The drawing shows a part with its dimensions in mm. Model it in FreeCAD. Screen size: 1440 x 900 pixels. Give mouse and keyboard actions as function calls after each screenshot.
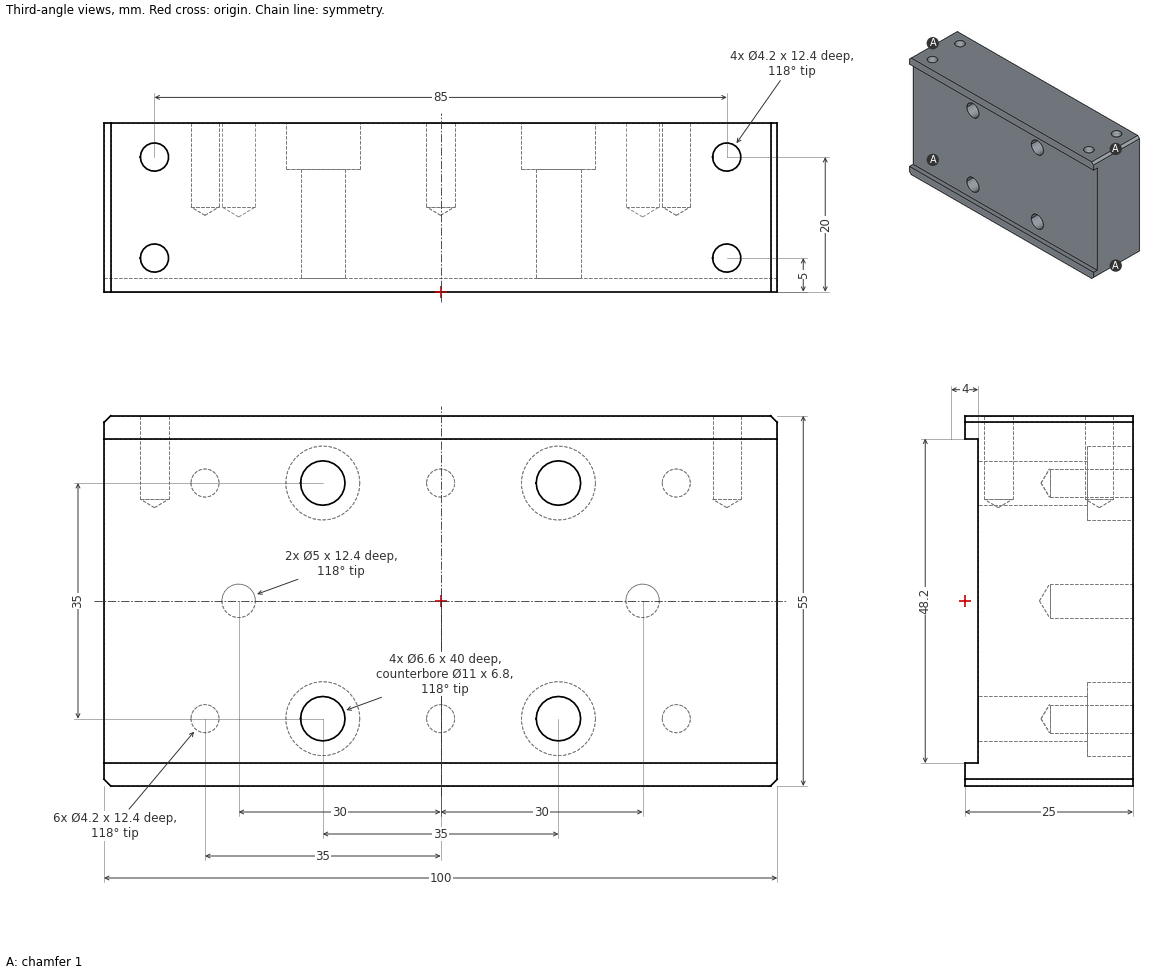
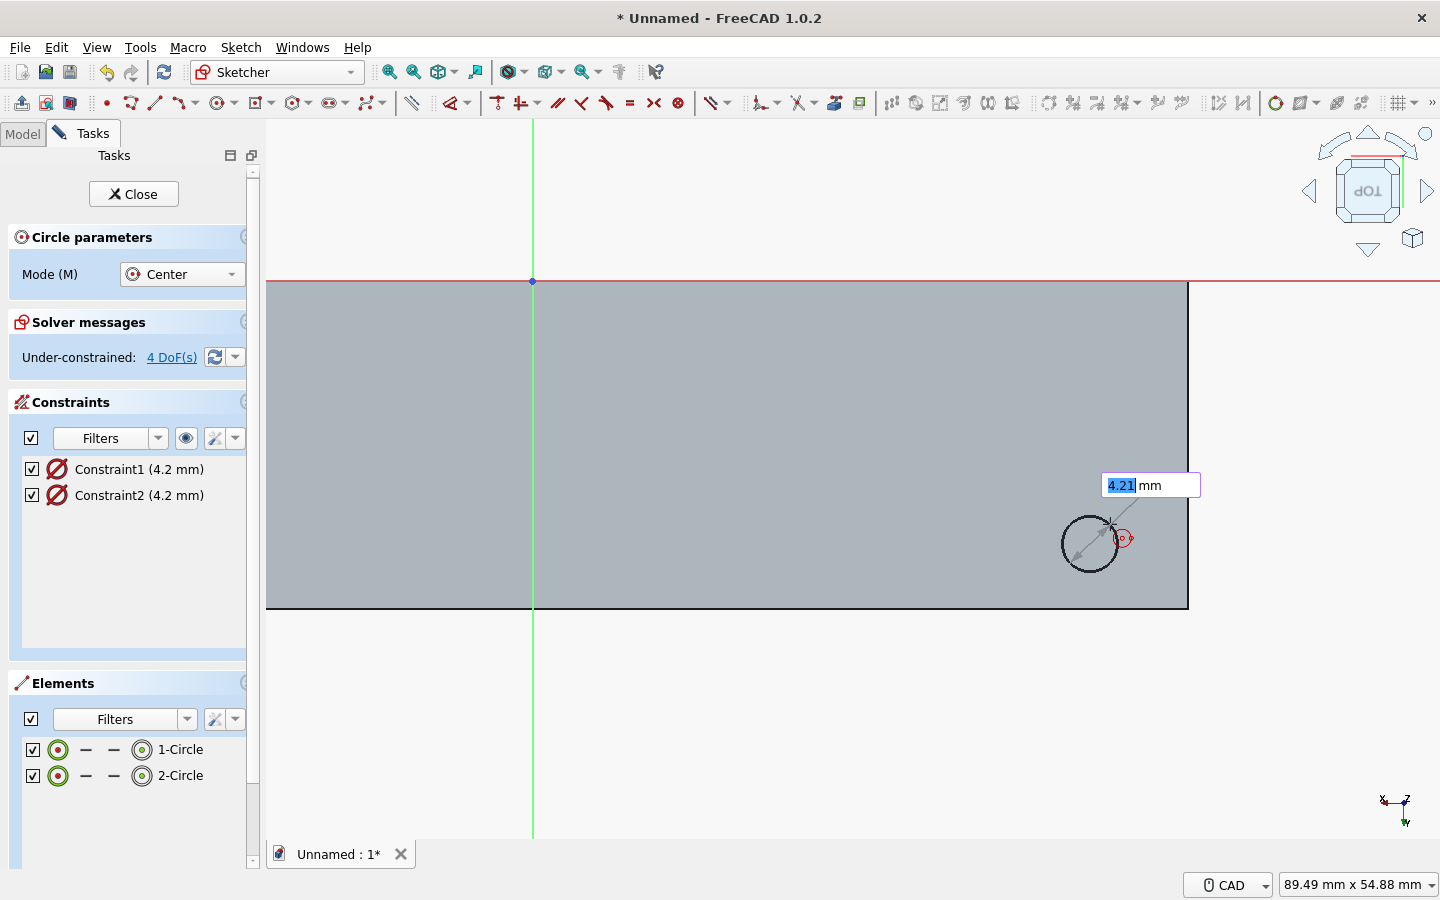
text(4.2)
key(Return)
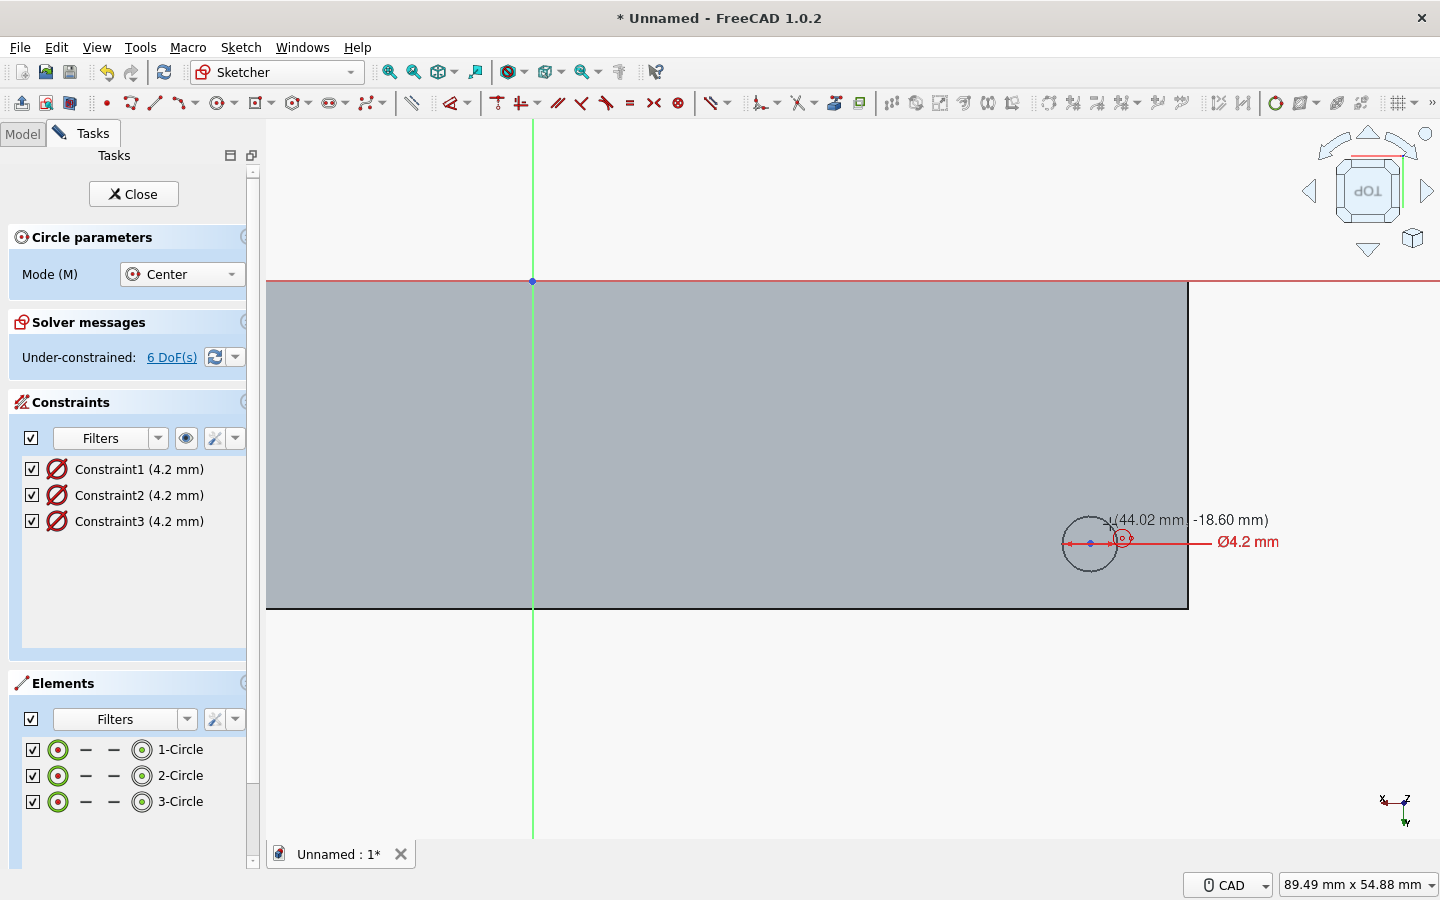
click(1090, 347)
move(1110, 327)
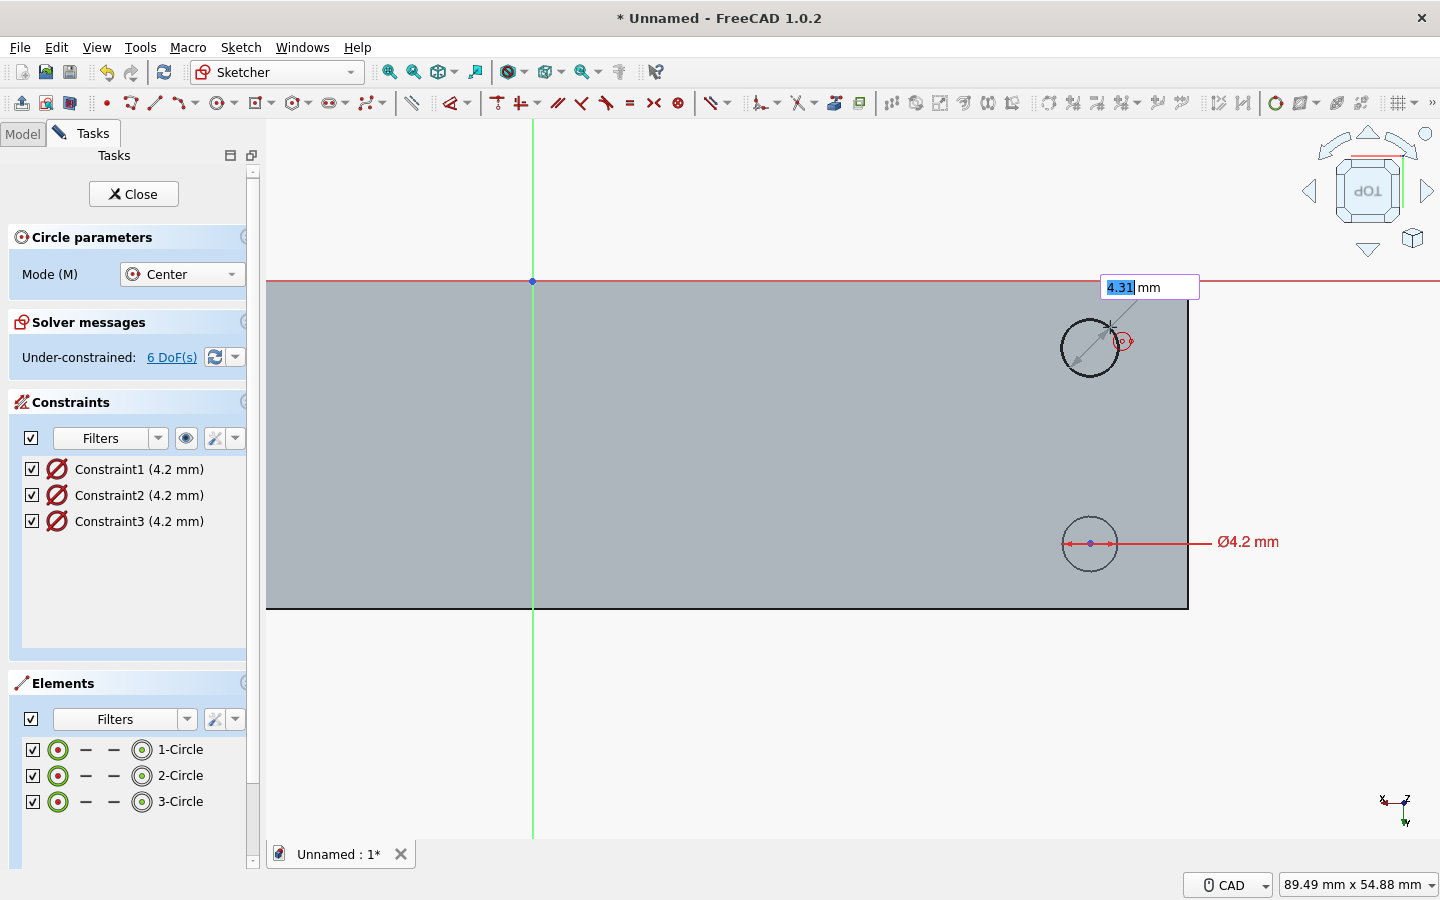
text(4.2)
key(Return)
key(Escape)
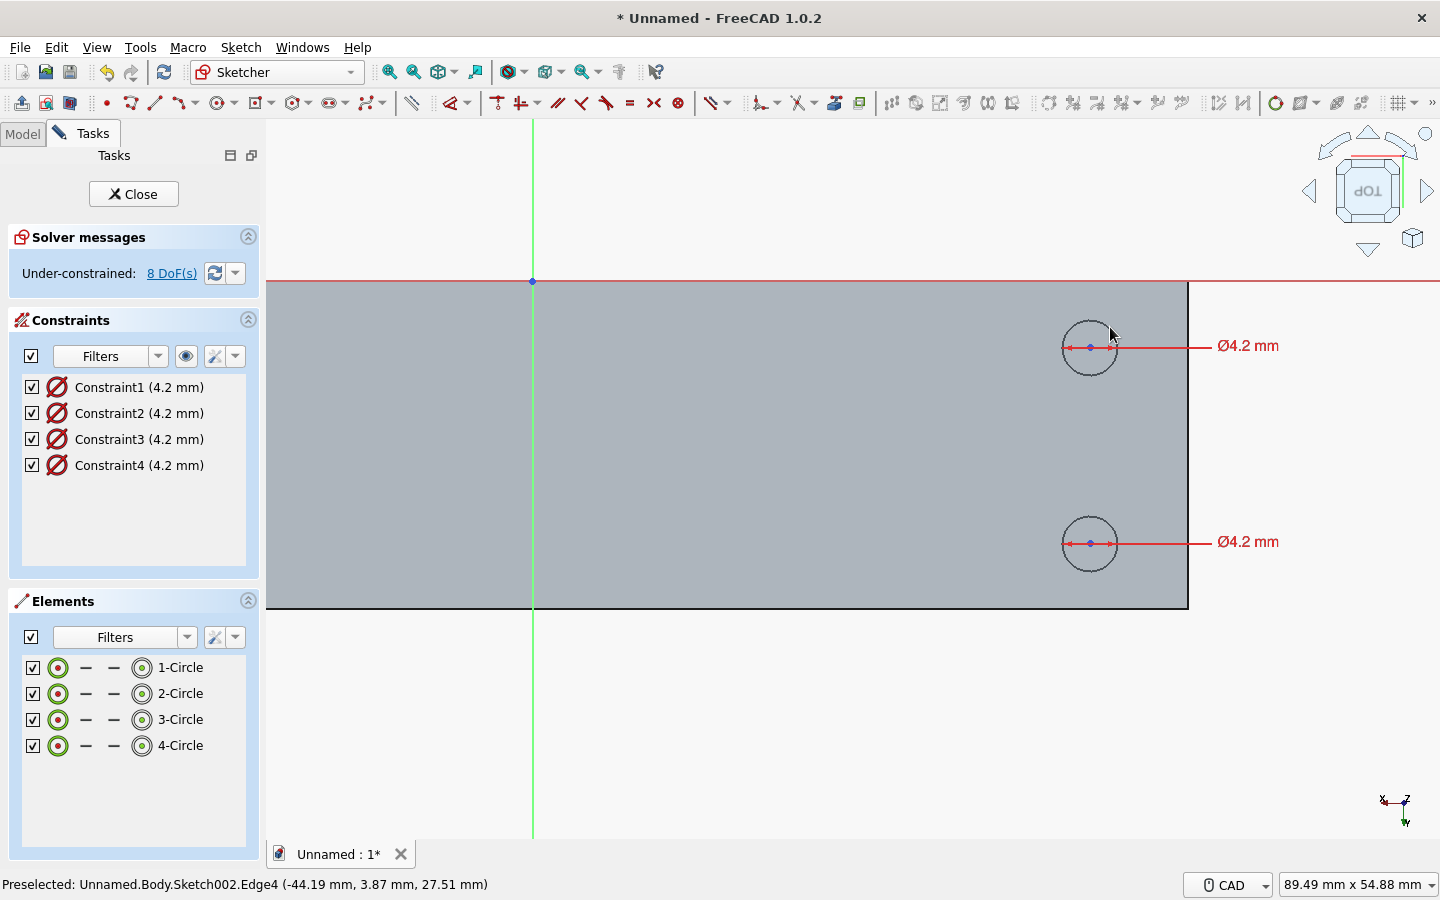
scroll(1091, 544, down, 3)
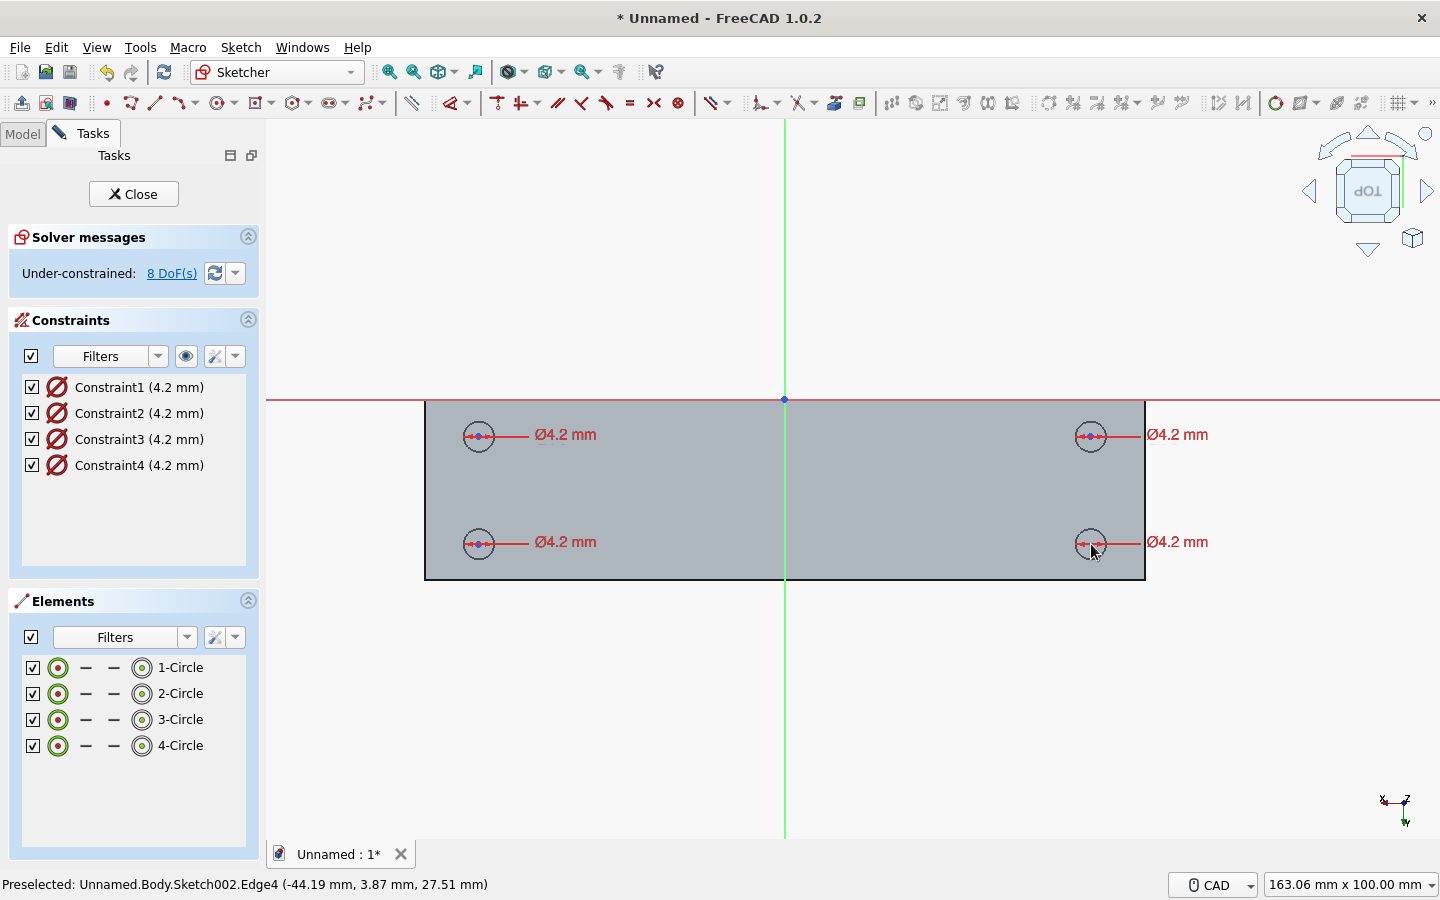
click(479, 544)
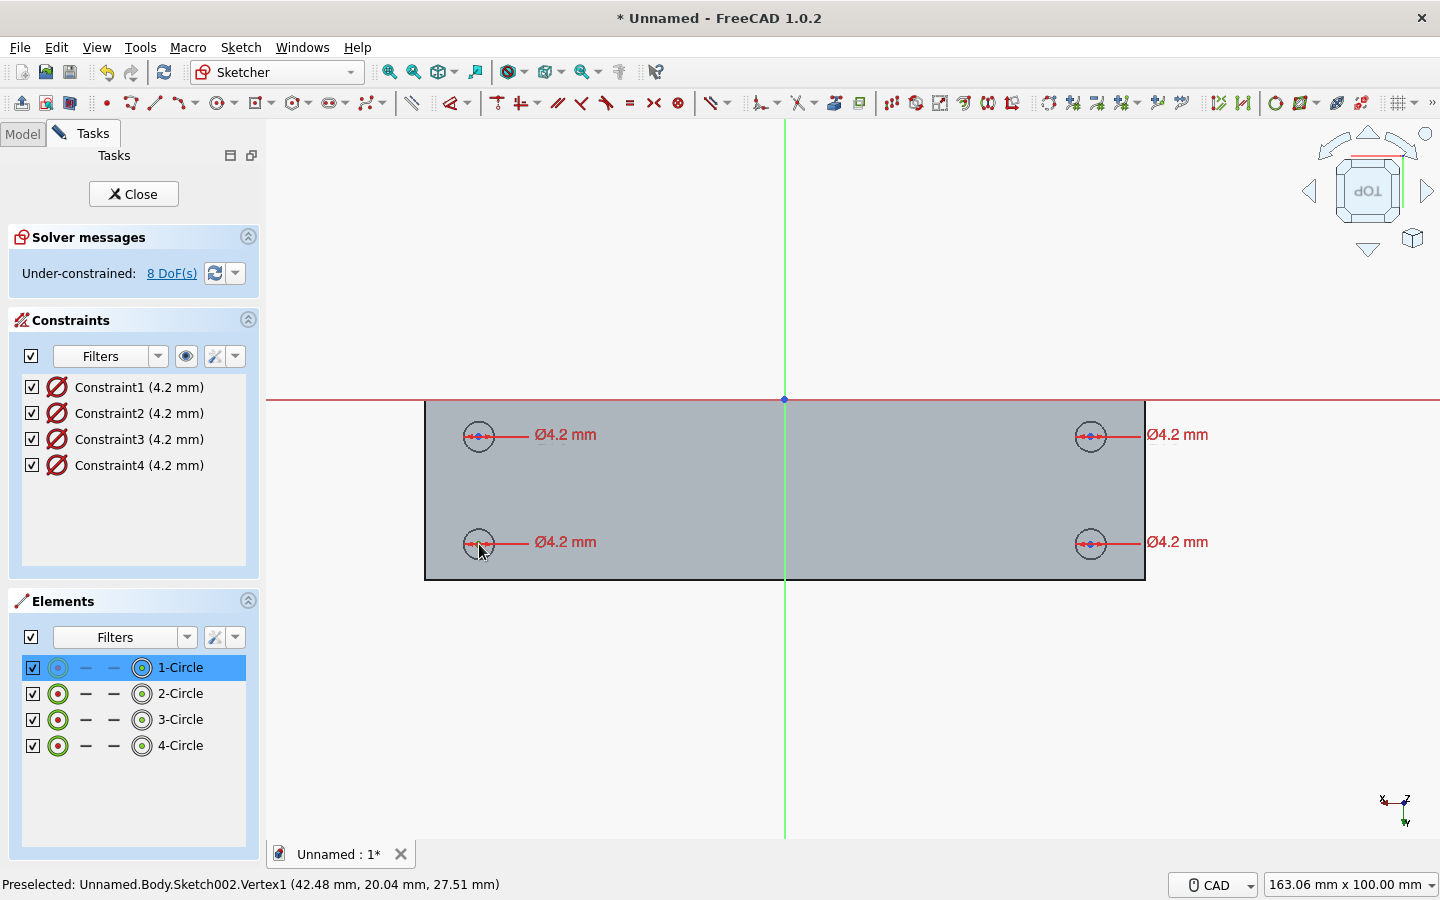
click(1091, 544)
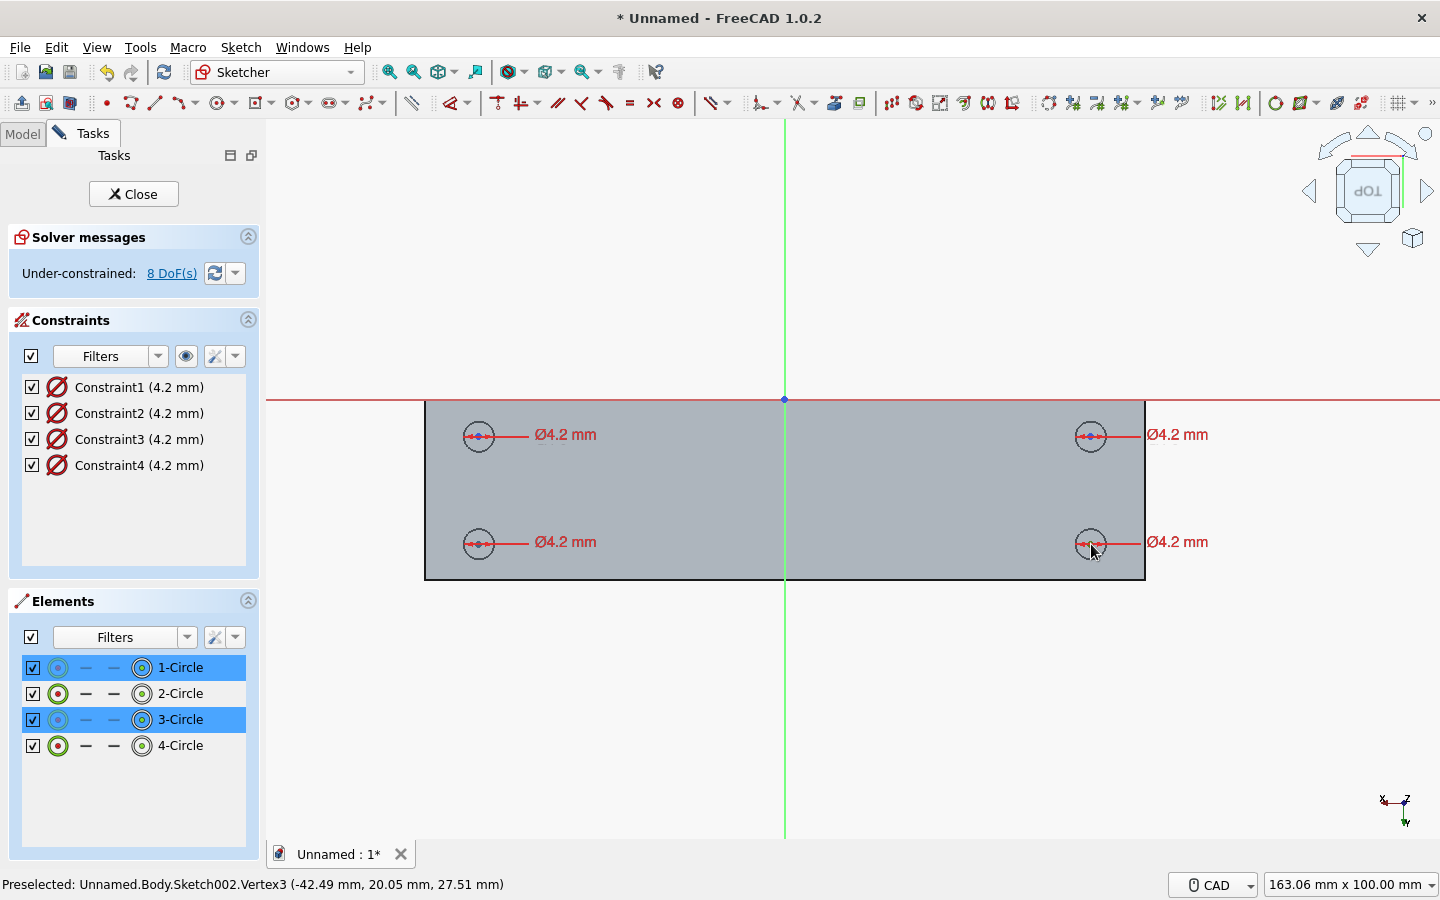
click(785, 764)